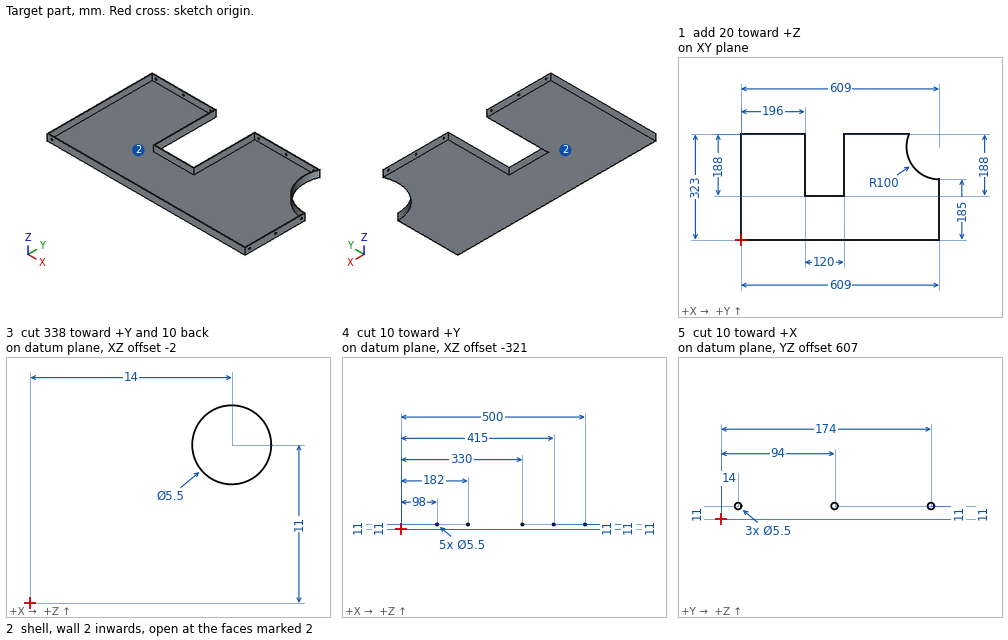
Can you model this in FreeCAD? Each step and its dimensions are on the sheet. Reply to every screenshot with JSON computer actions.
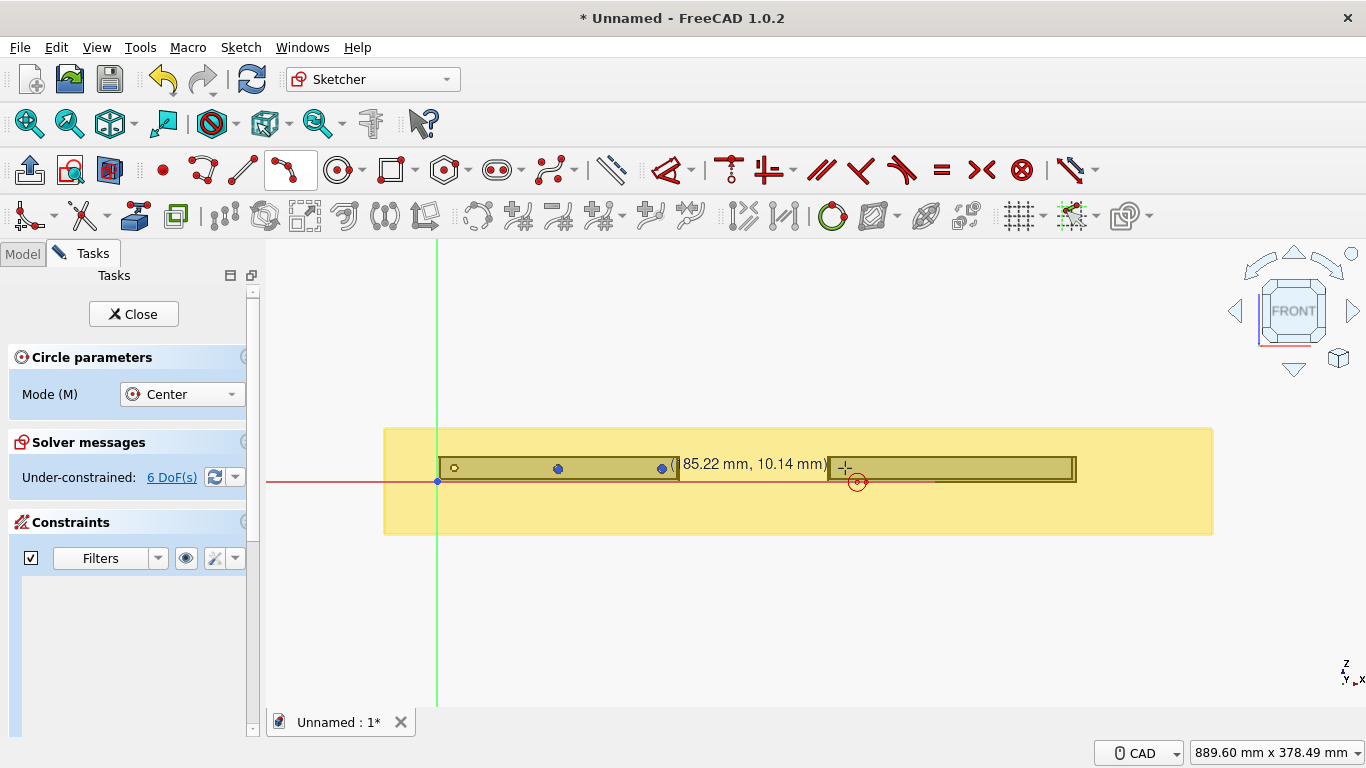
{"action": "left_click", "coordinate": [845, 468]}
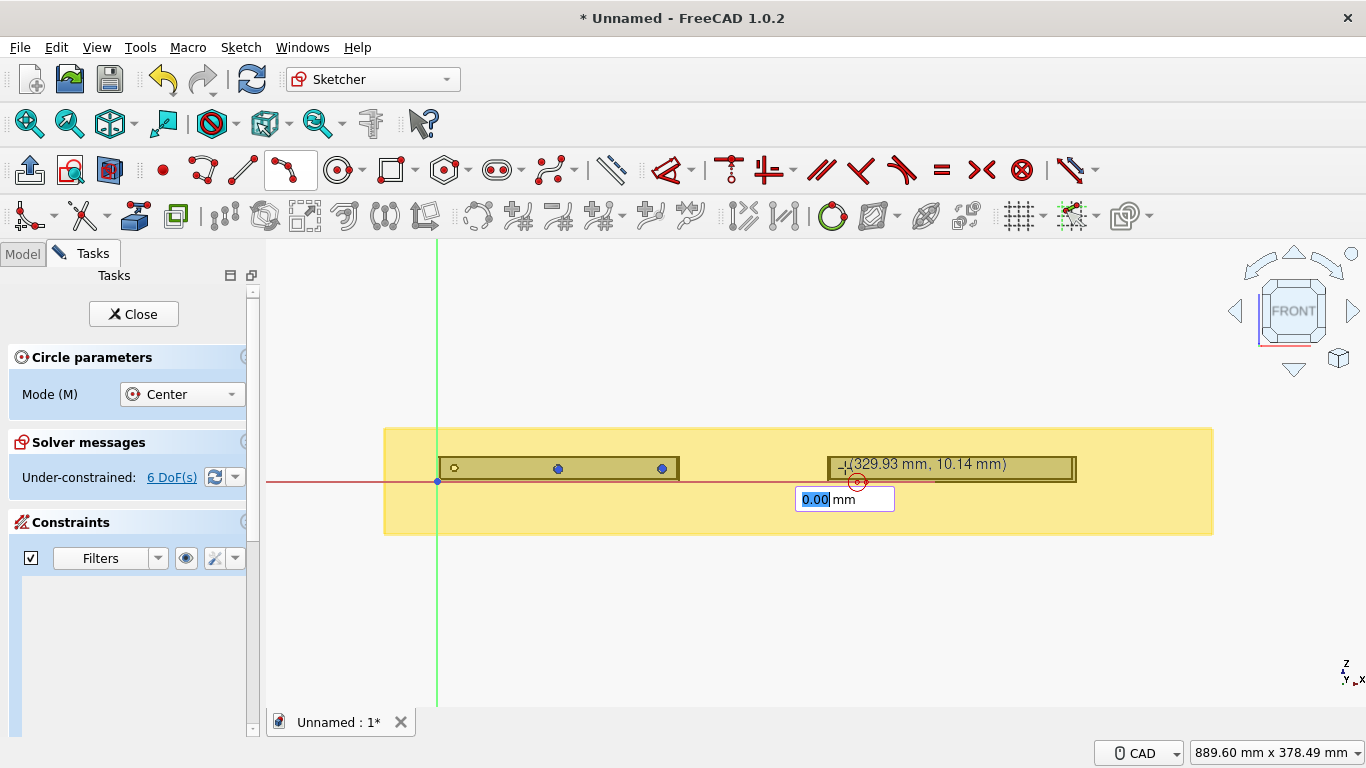
{"action": "scroll", "coordinate": [847, 466], "scroll_direction": "up", "scroll_amount": 8}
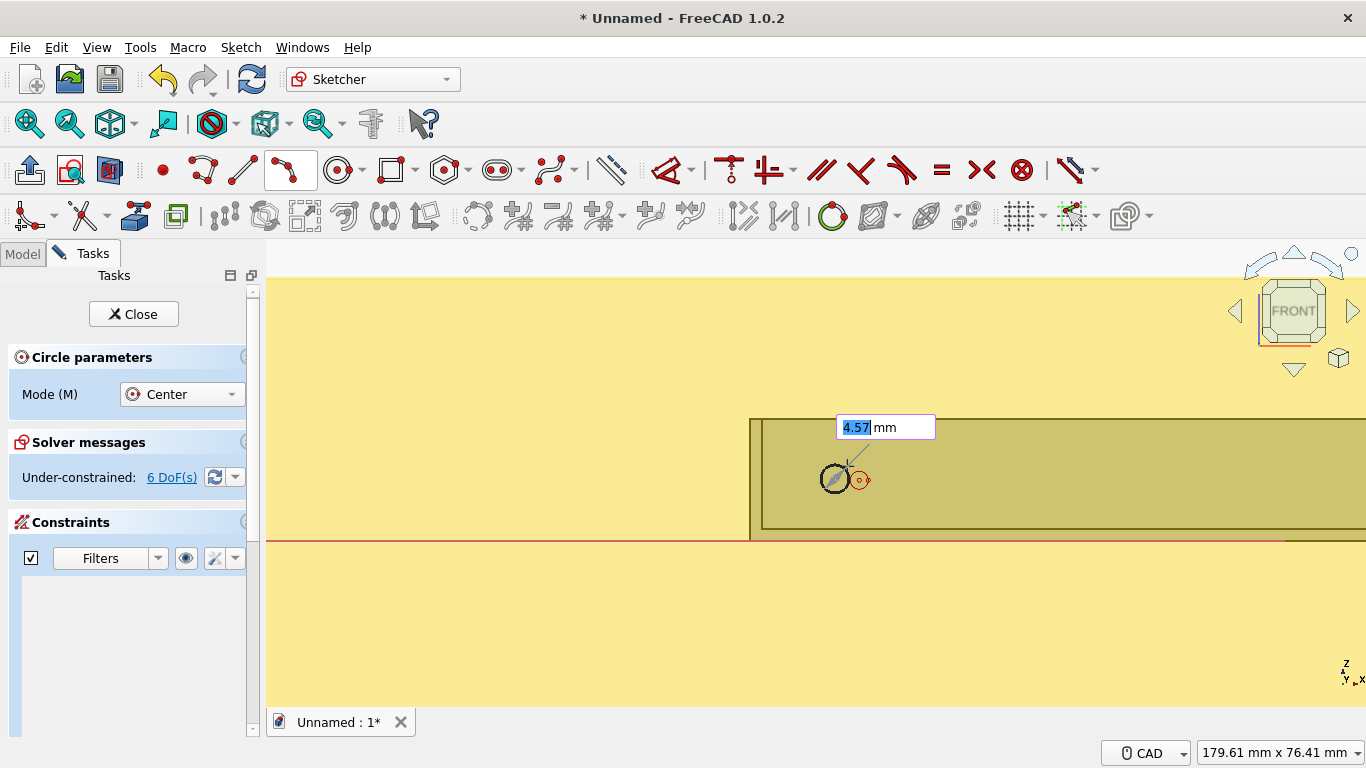
{"action": "left_click", "coordinate": [847, 462]}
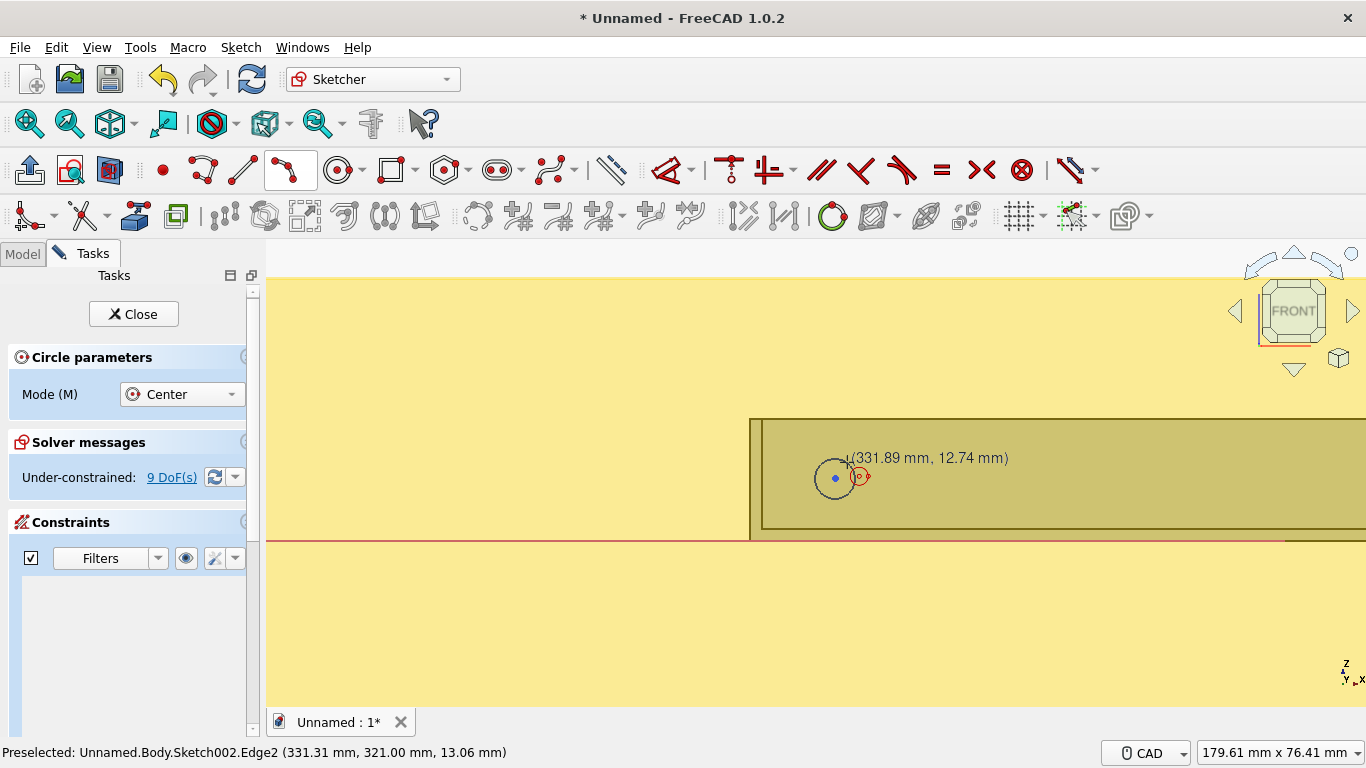
{"action": "scroll", "coordinate": [847, 466], "scroll_direction": "down", "scroll_amount": 8}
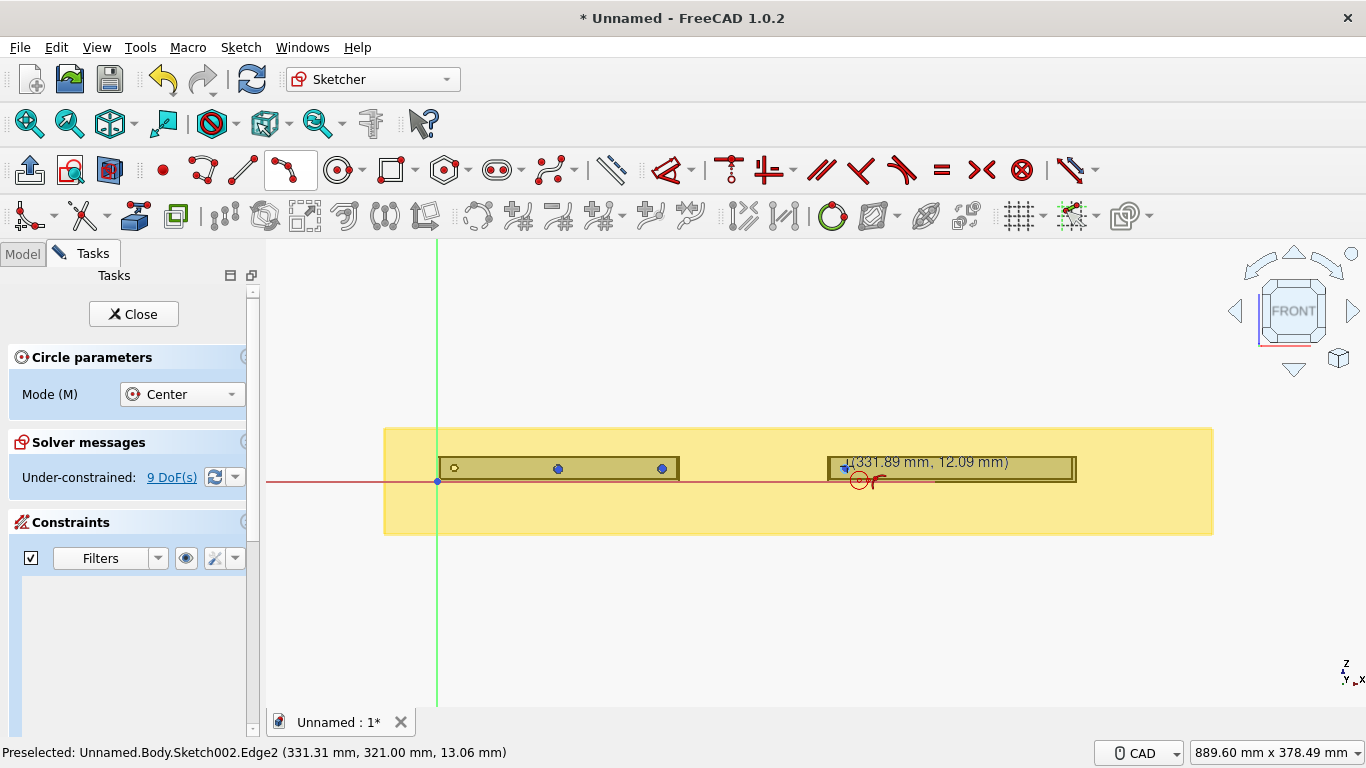
{"action": "scroll", "coordinate": [950, 468], "scroll_direction": "up", "scroll_amount": 10}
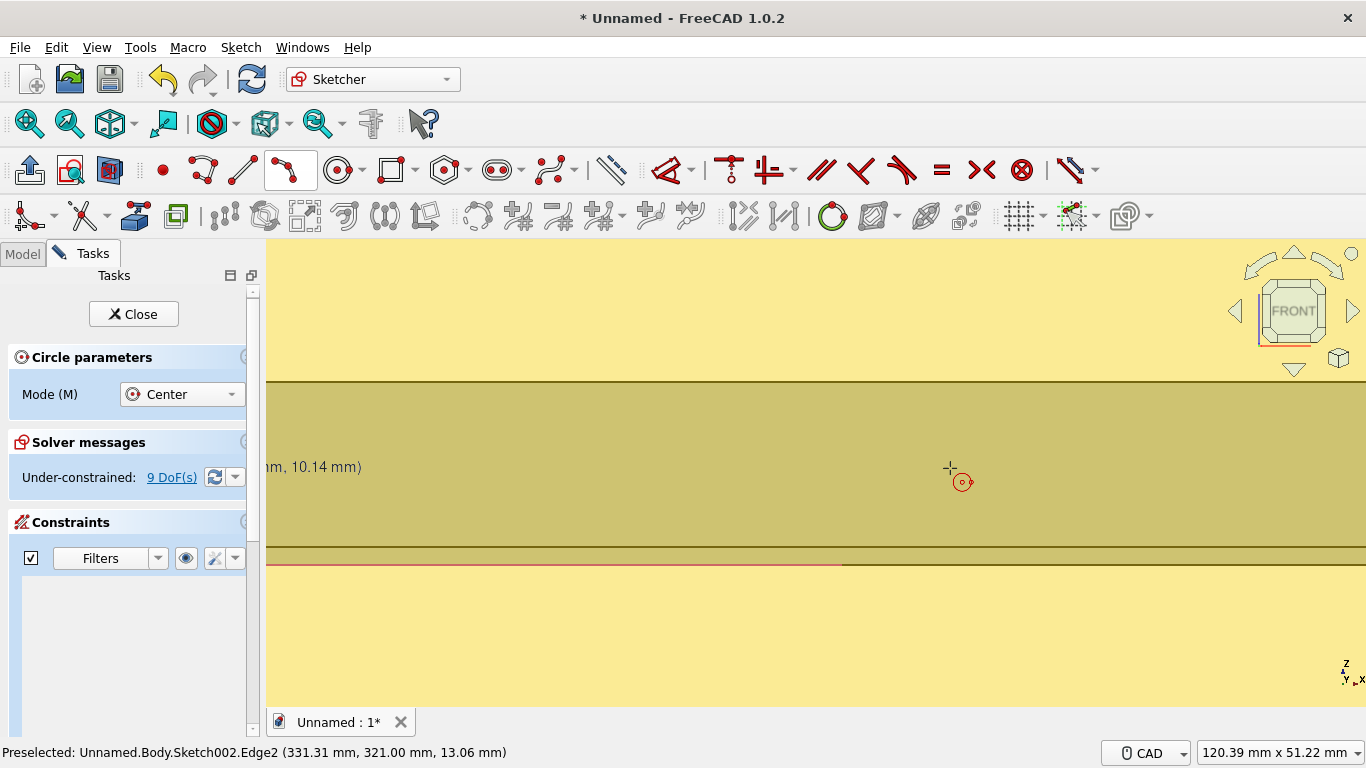
{"action": "scroll", "coordinate": [950, 468], "scroll_direction": "down", "scroll_amount": 10}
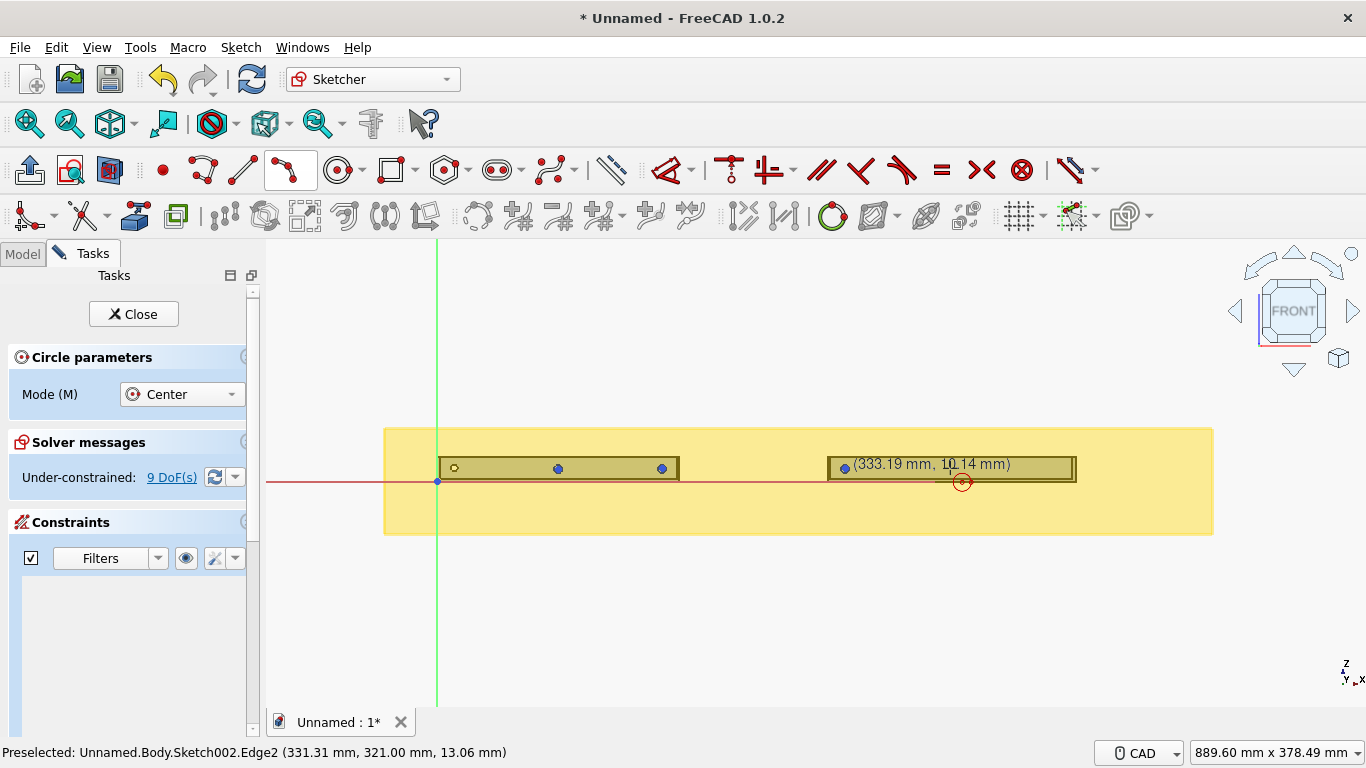
{"action": "left_click", "coordinate": [950, 468]}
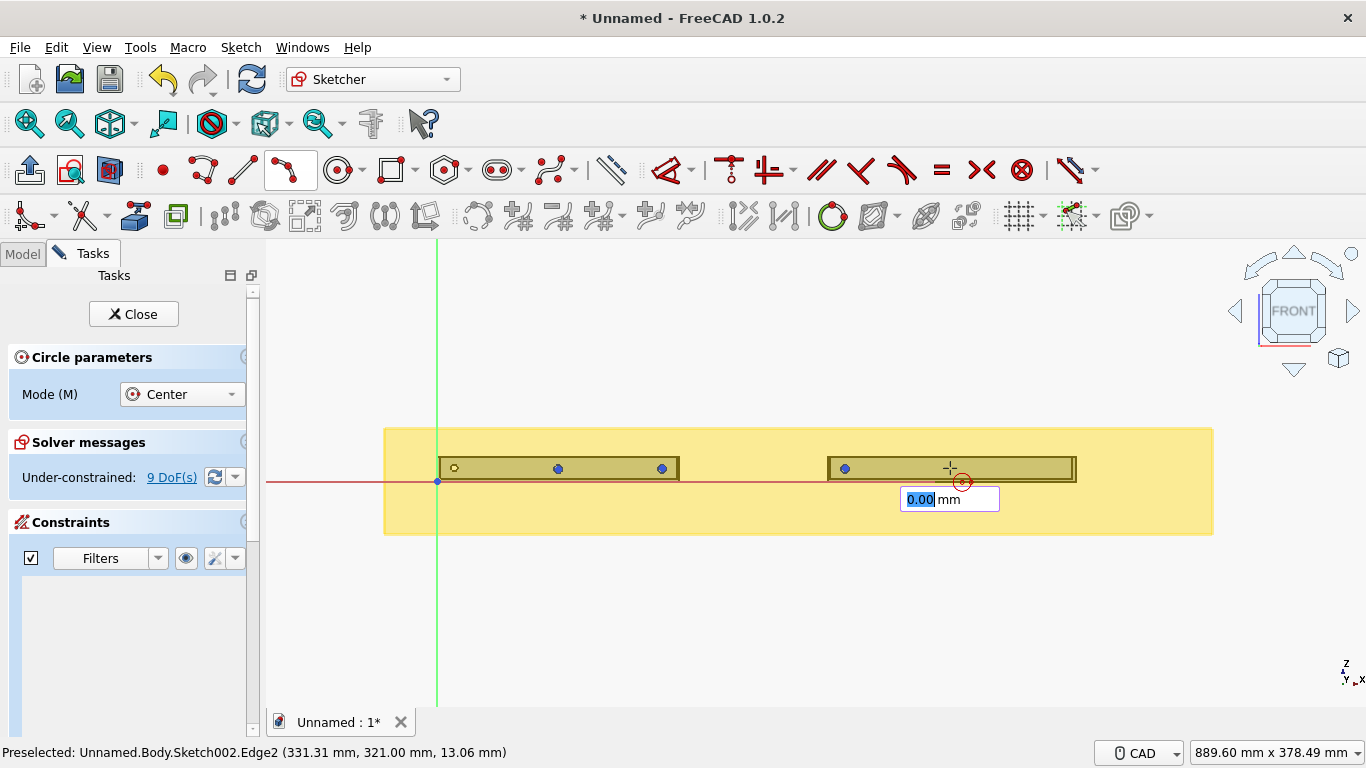
{"action": "scroll", "coordinate": [953, 466], "scroll_direction": "up", "scroll_amount": 8}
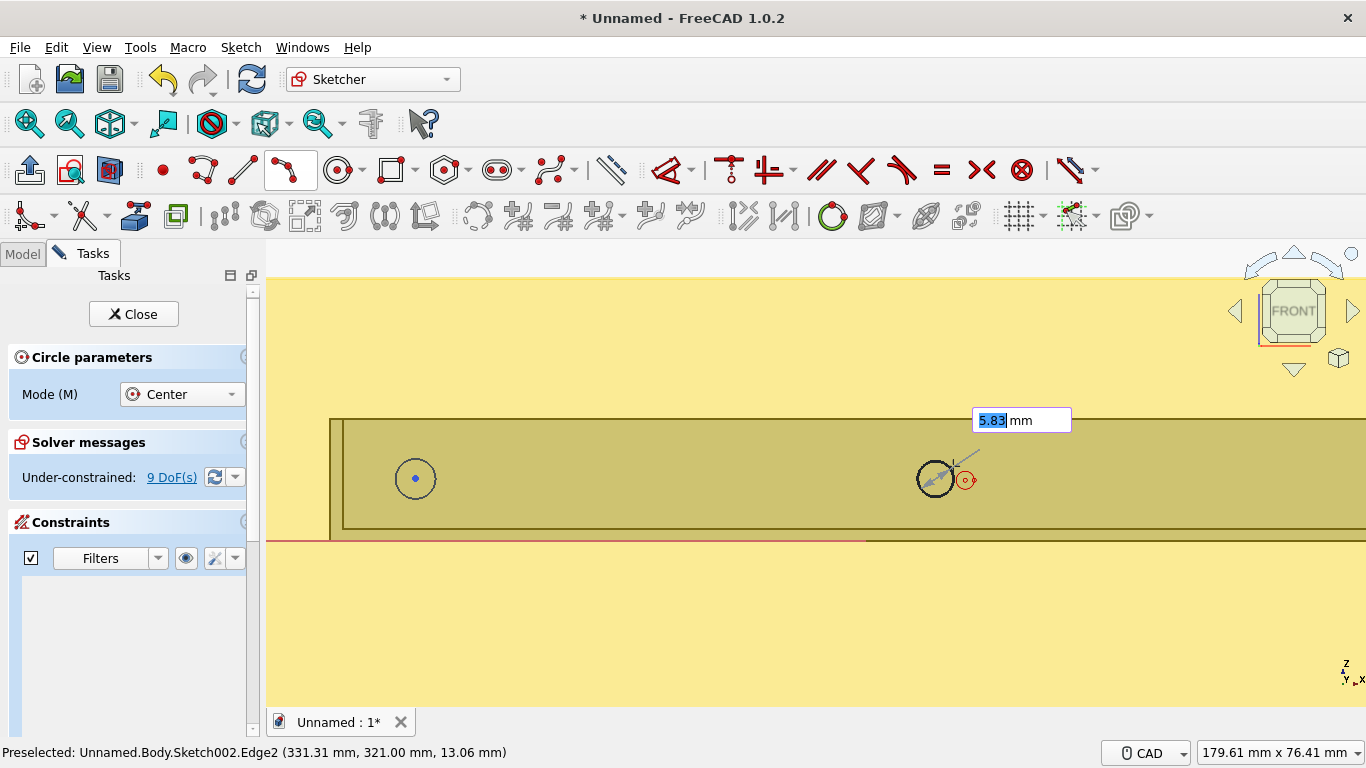
{"action": "left_click", "coordinate": [949, 462]}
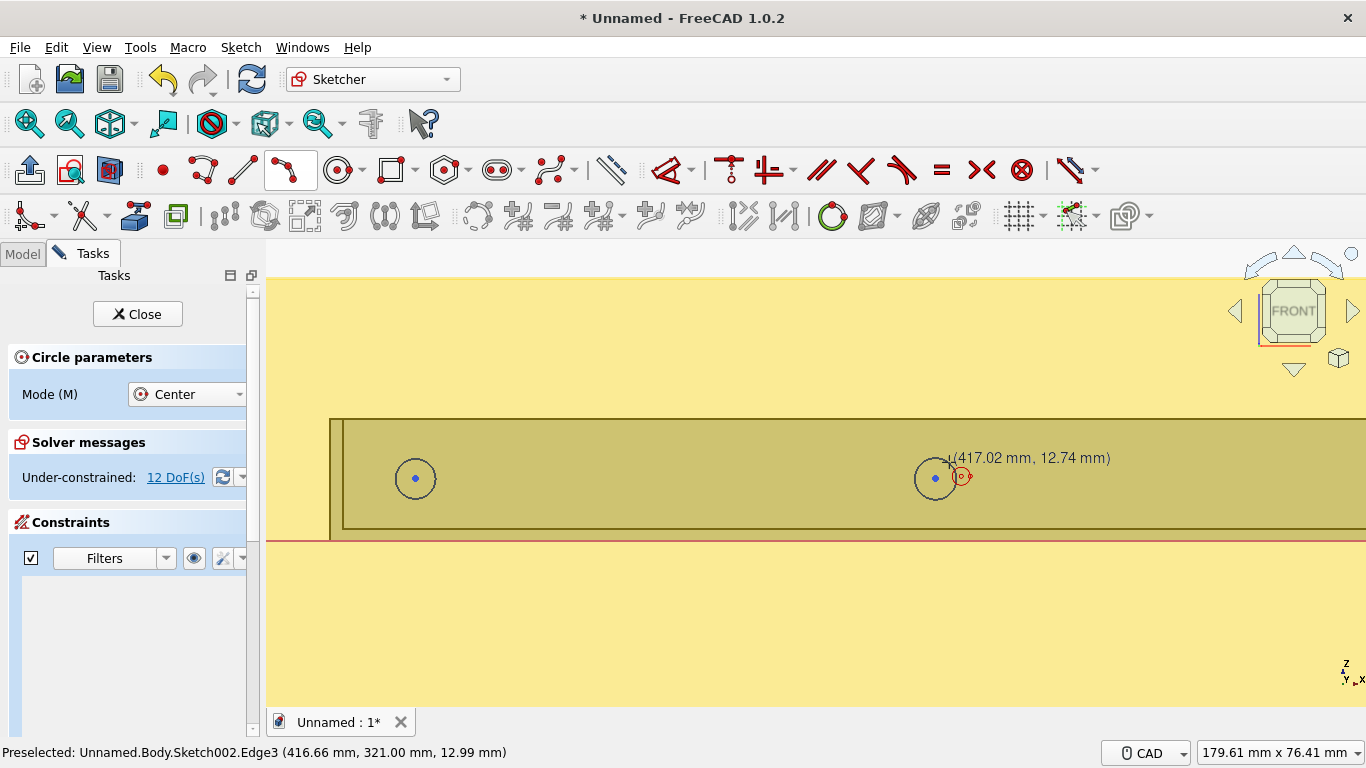
{"action": "scroll", "coordinate": [953, 466], "scroll_direction": "down", "scroll_amount": 8}